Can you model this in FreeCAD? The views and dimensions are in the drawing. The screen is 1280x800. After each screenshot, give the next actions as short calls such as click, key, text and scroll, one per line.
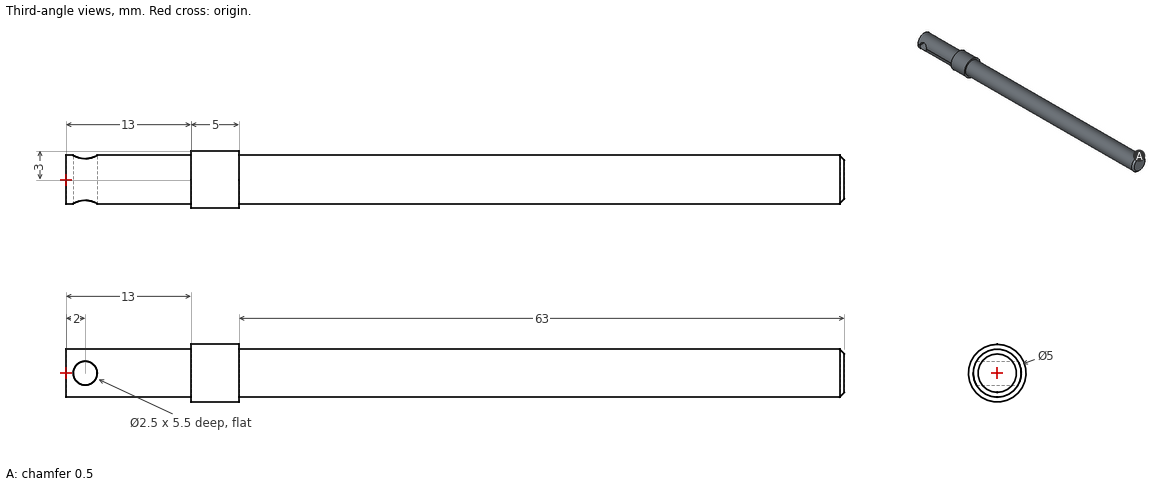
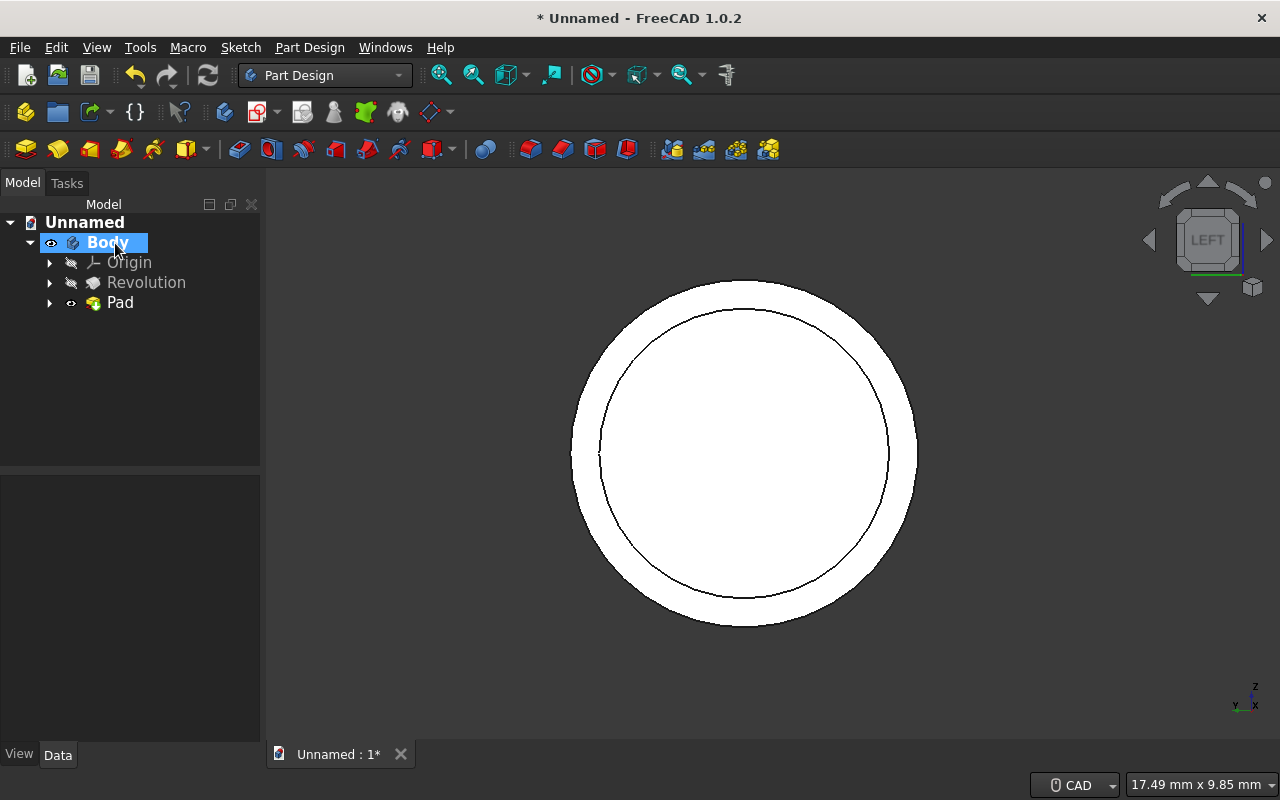
click(50, 263)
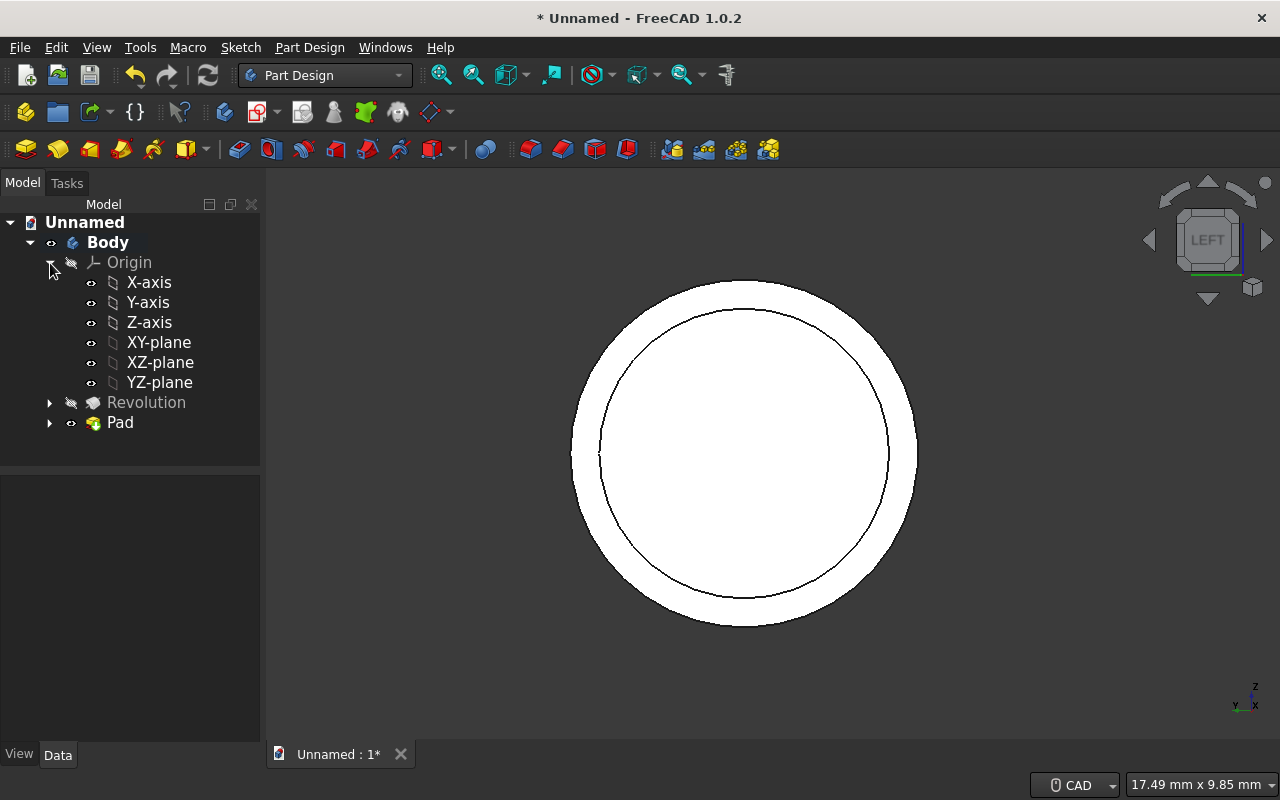
click(136, 383)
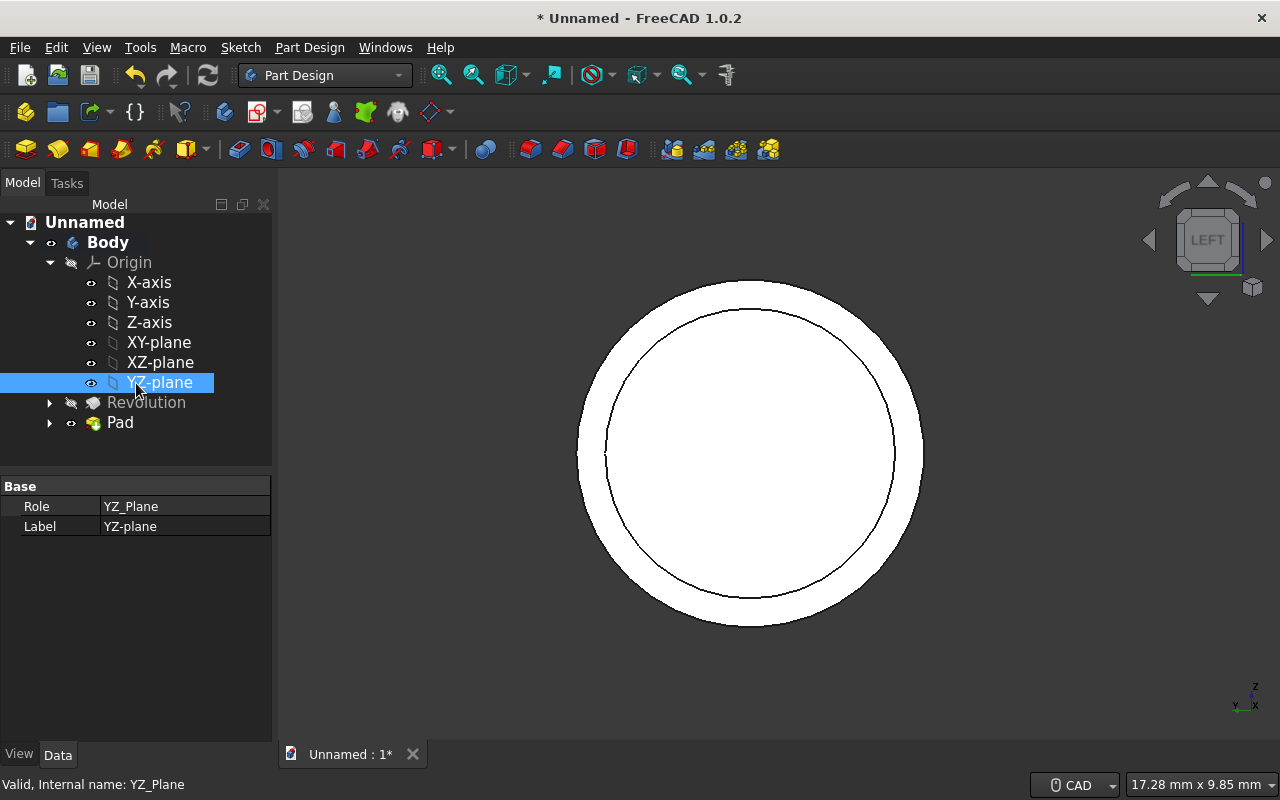
click(430, 112)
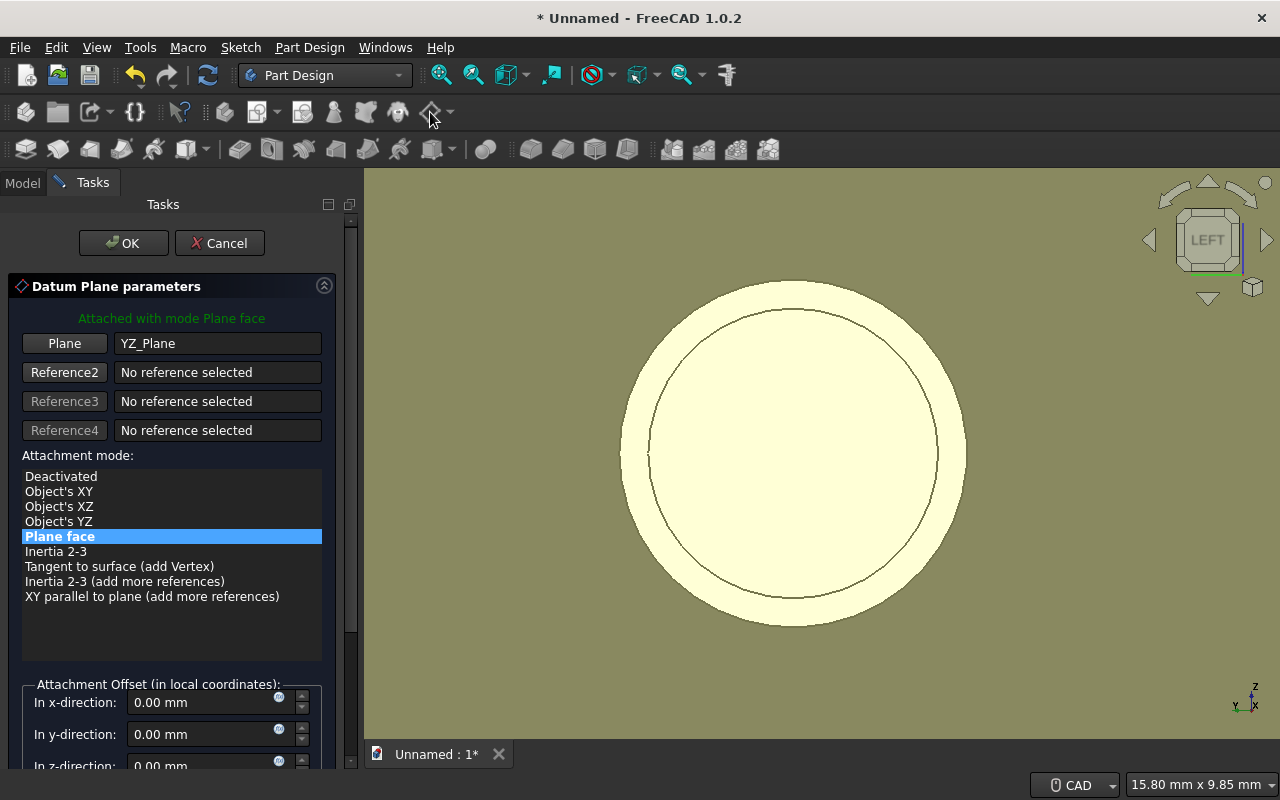
scroll(351, 491, down, 2)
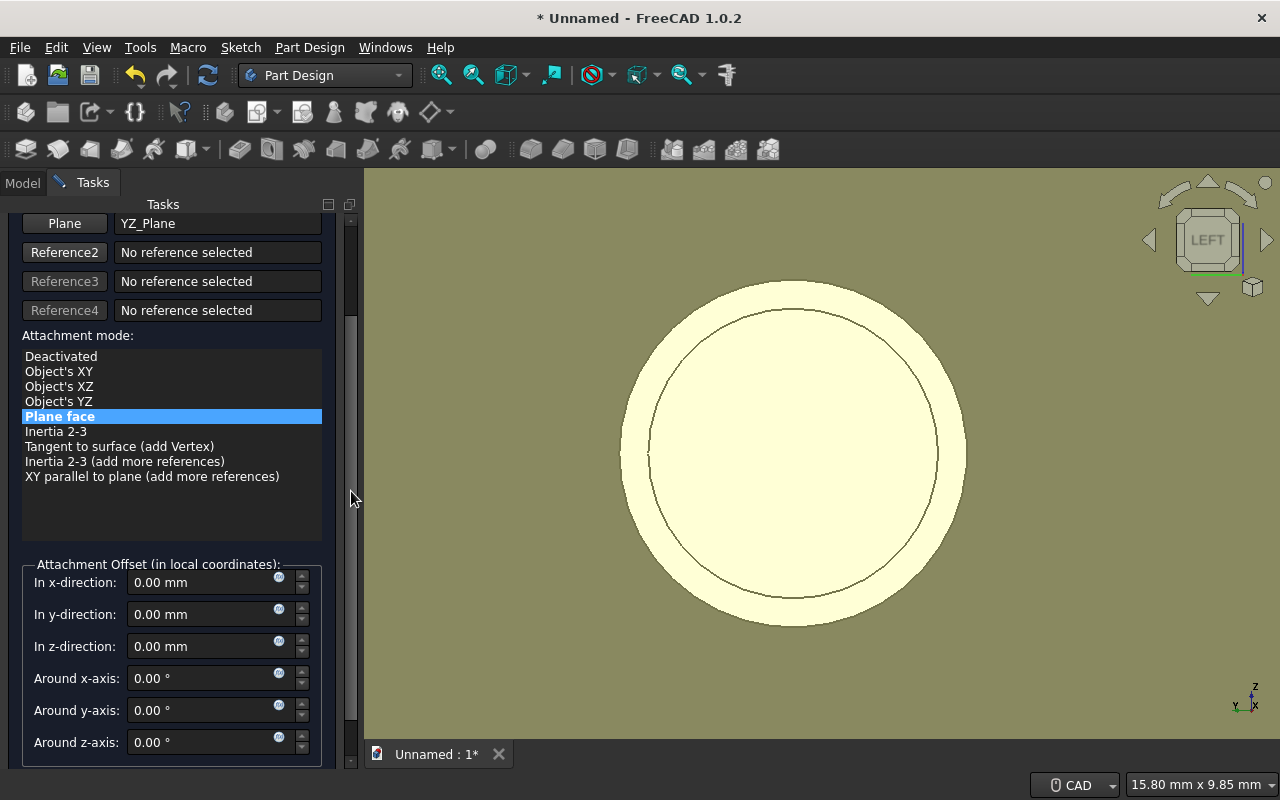
triple_click(210, 646)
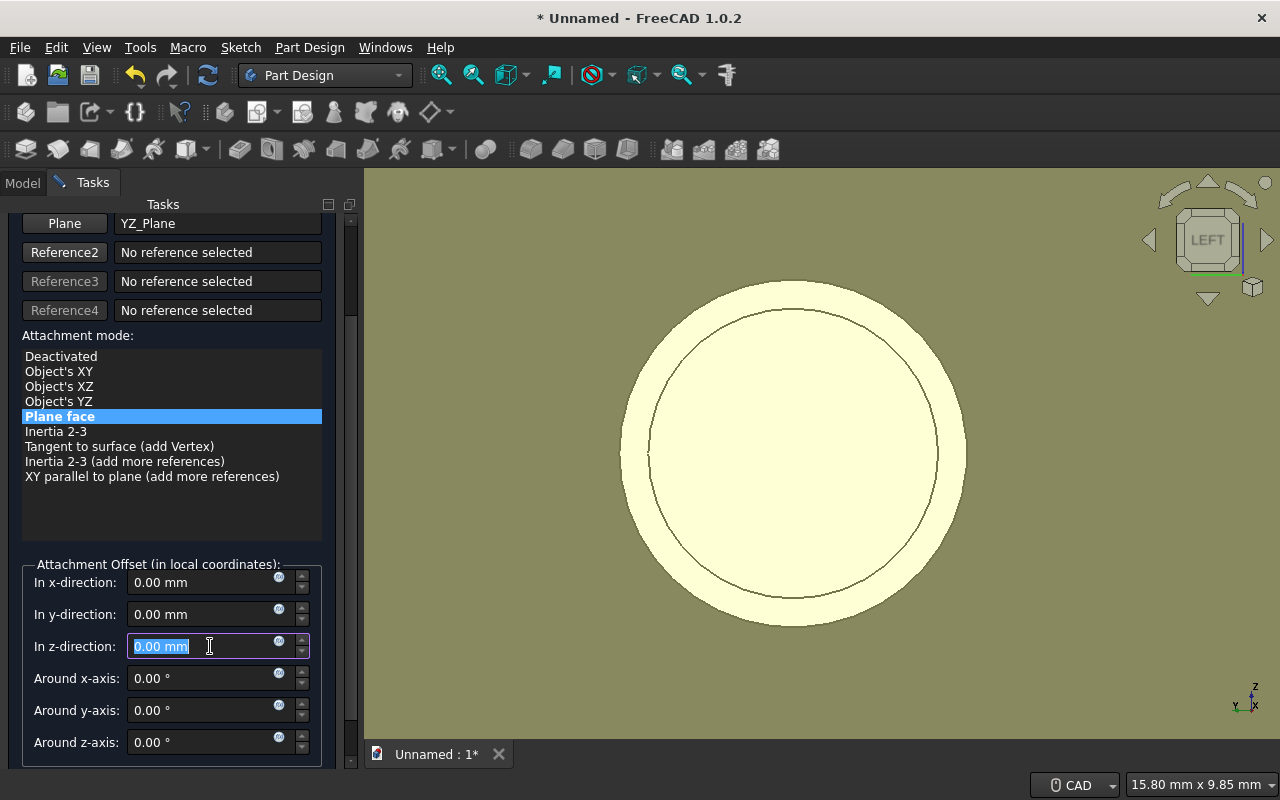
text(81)
key(Tab)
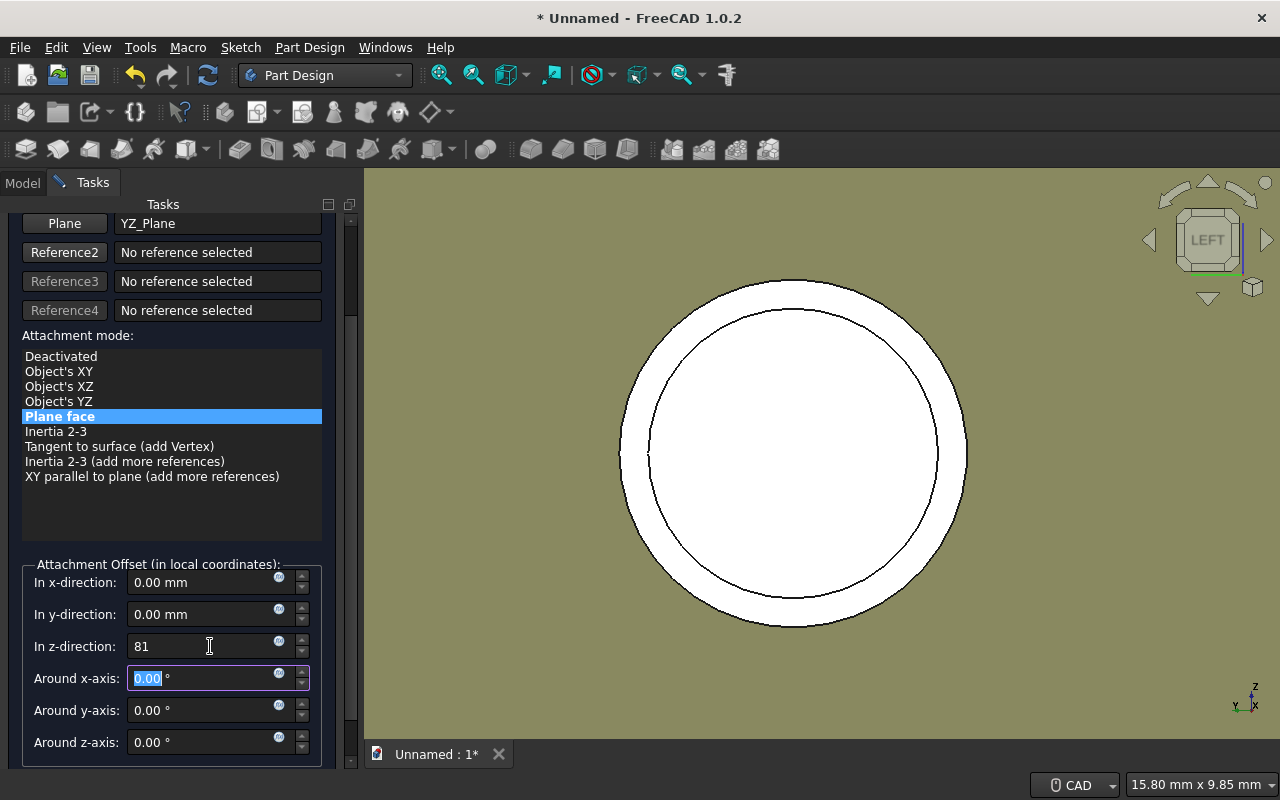
scroll(351, 491, up, 3)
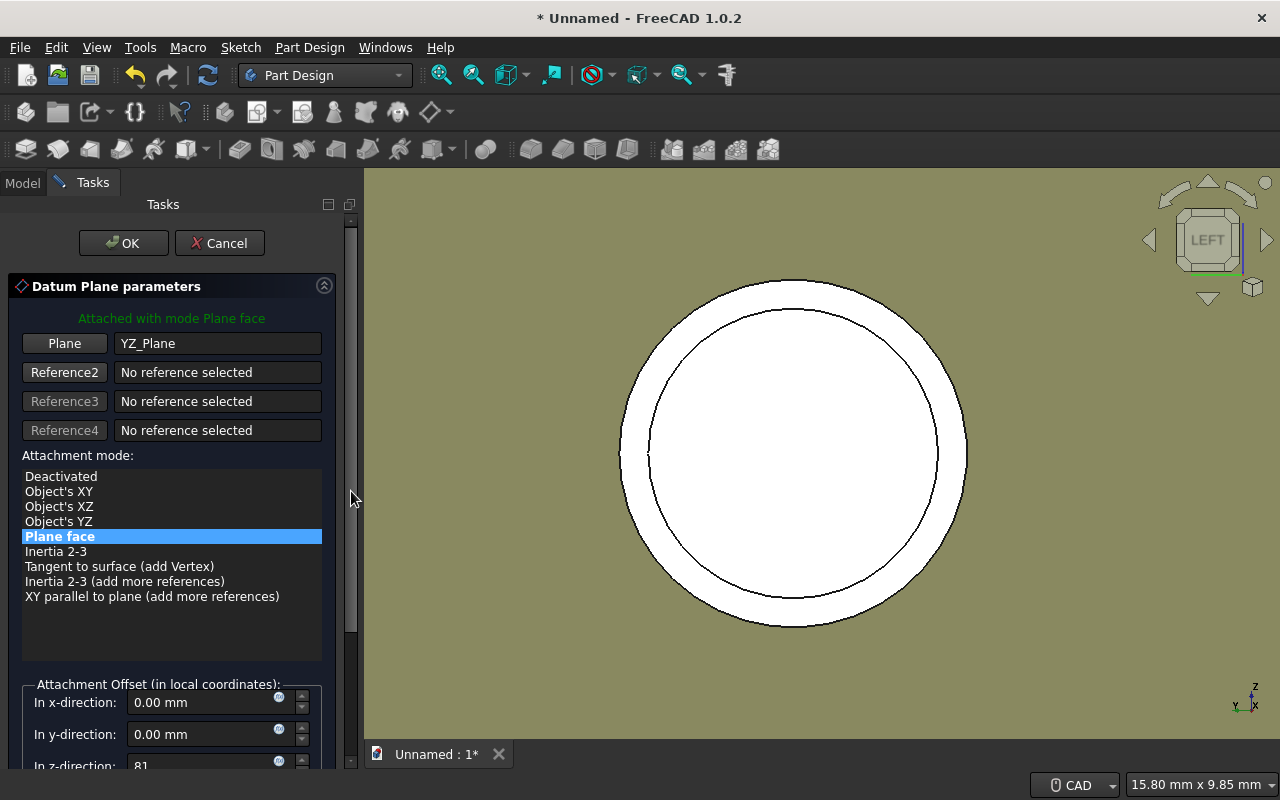
click(124, 243)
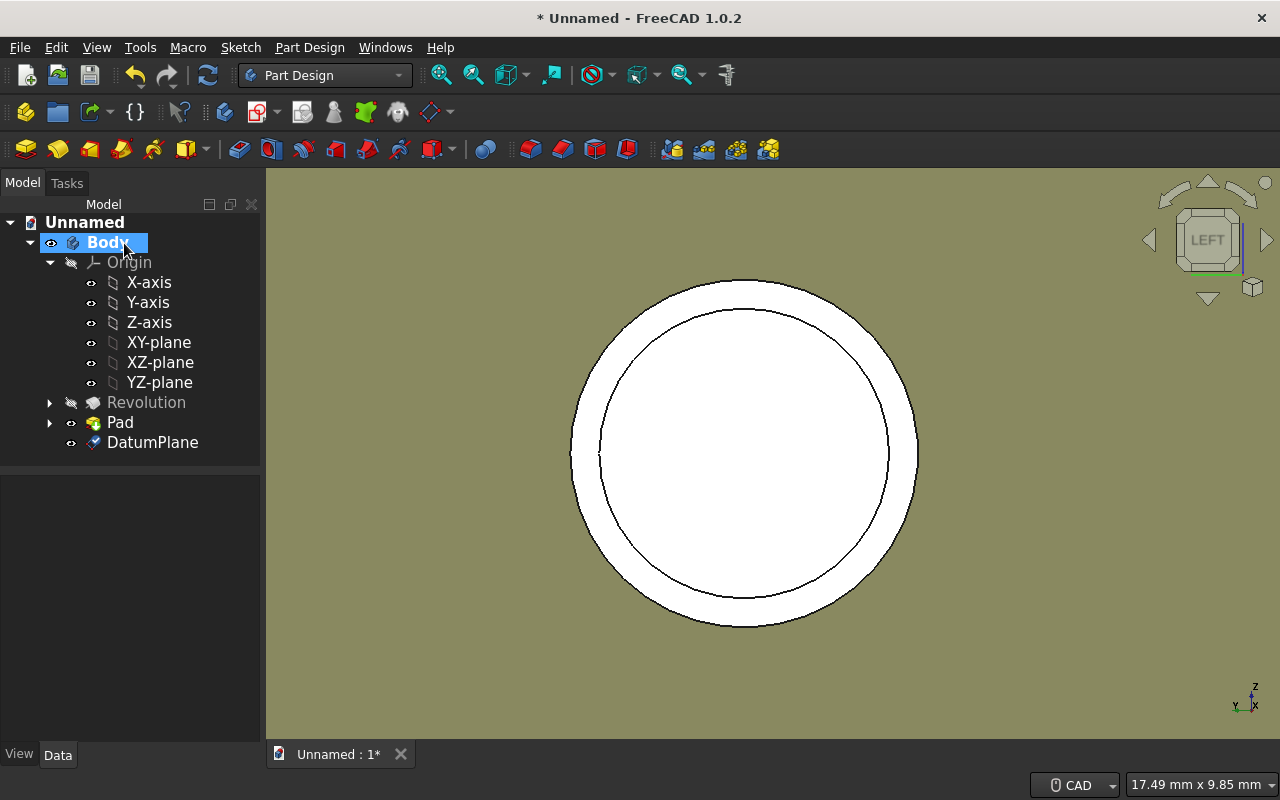
click(116, 443)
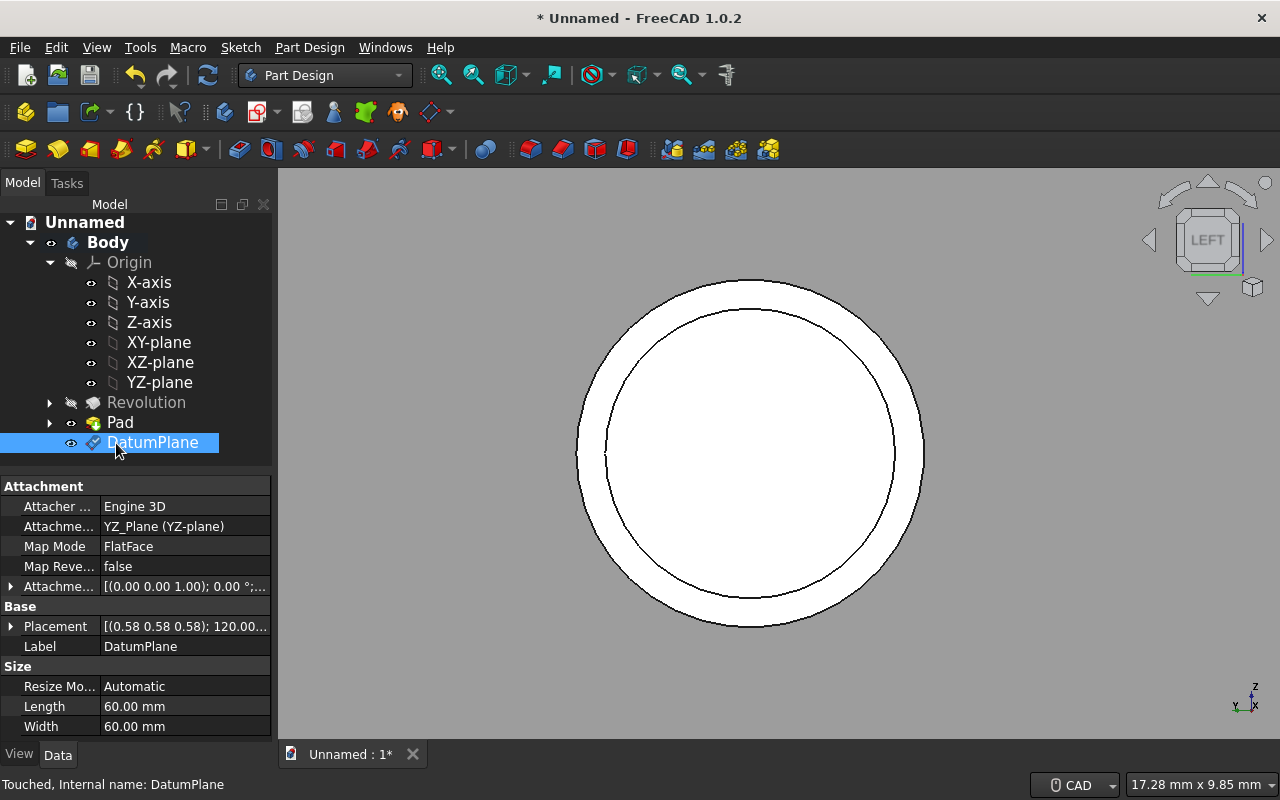
click(258, 112)